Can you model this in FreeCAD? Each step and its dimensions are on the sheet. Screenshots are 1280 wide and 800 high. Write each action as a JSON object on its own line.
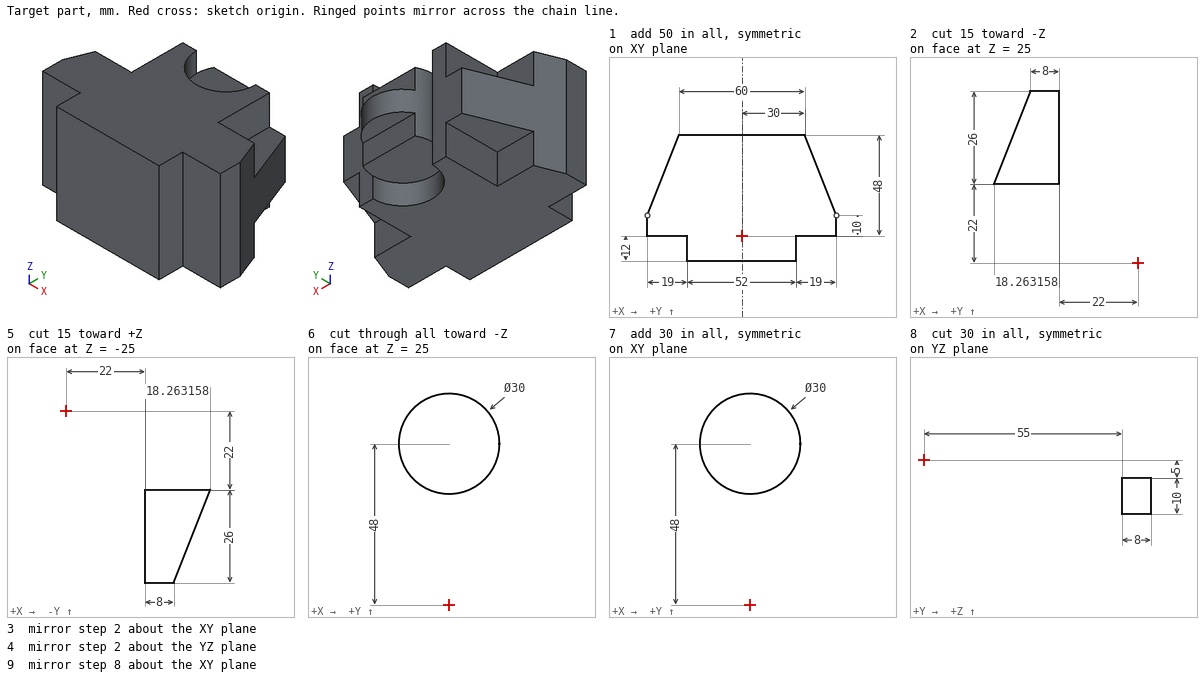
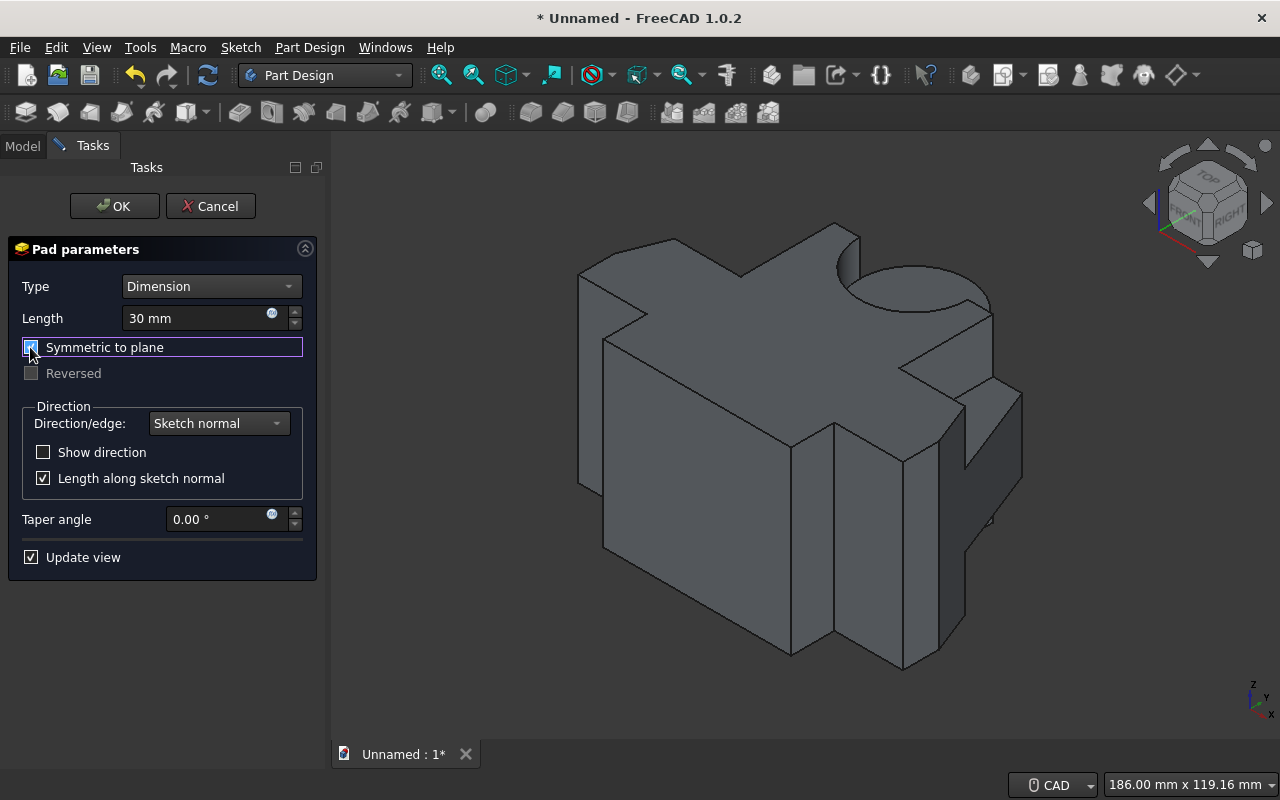
{"action": "left_click", "coordinate": [115, 206]}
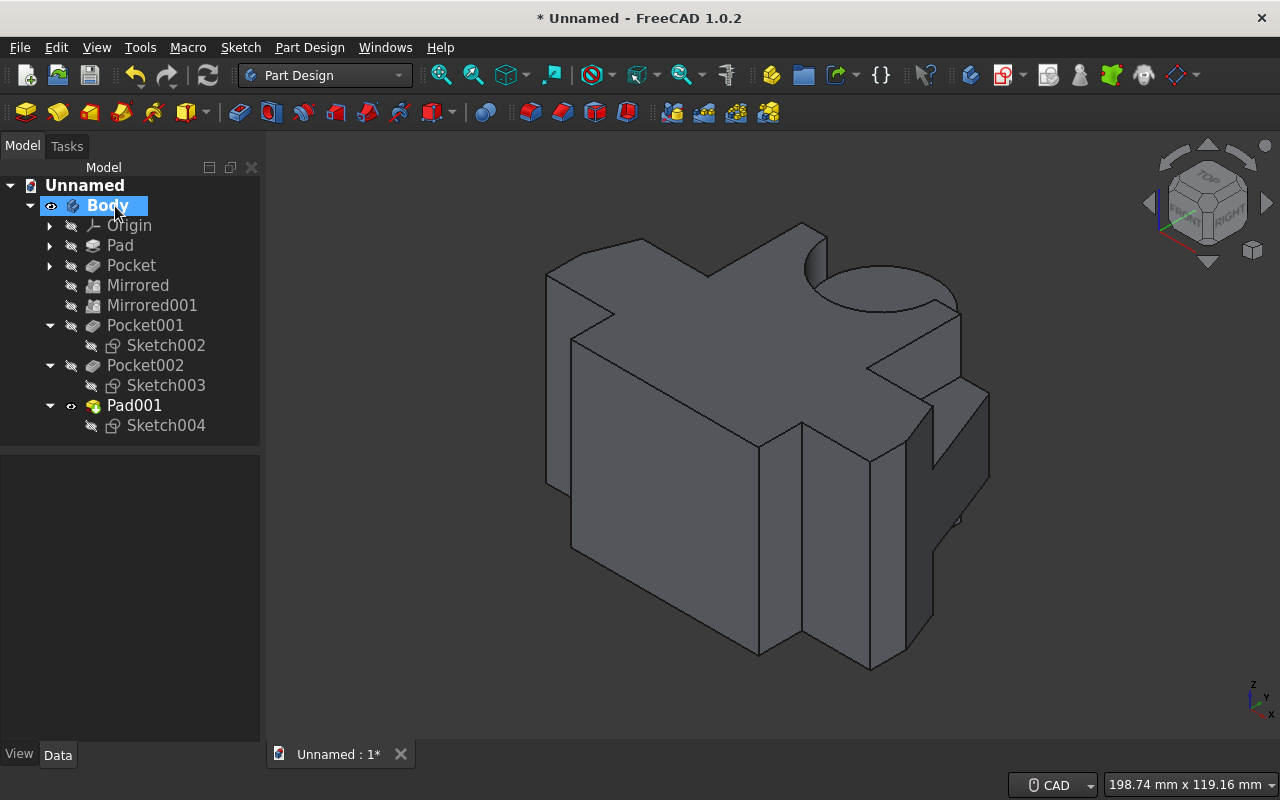
{"action": "left_click", "coordinate": [1004, 76]}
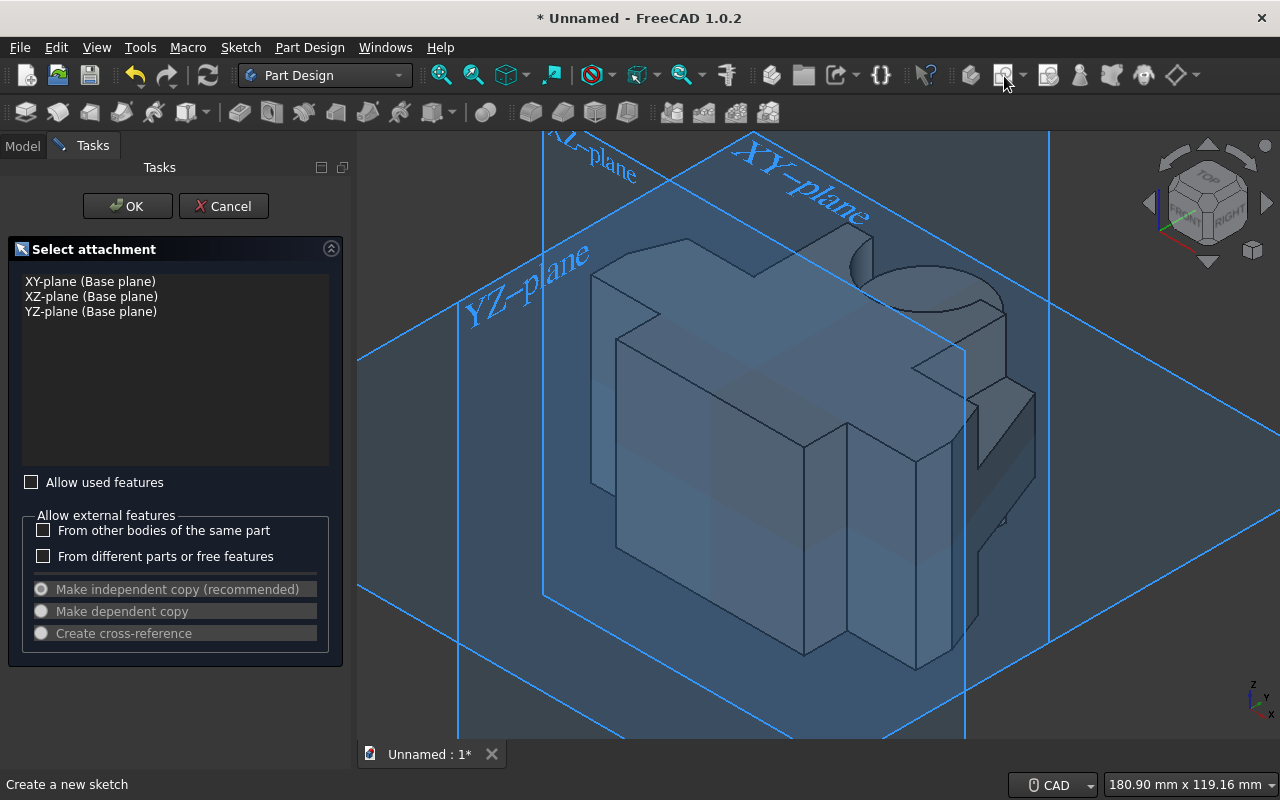
{"action": "left_click", "coordinate": [82, 312]}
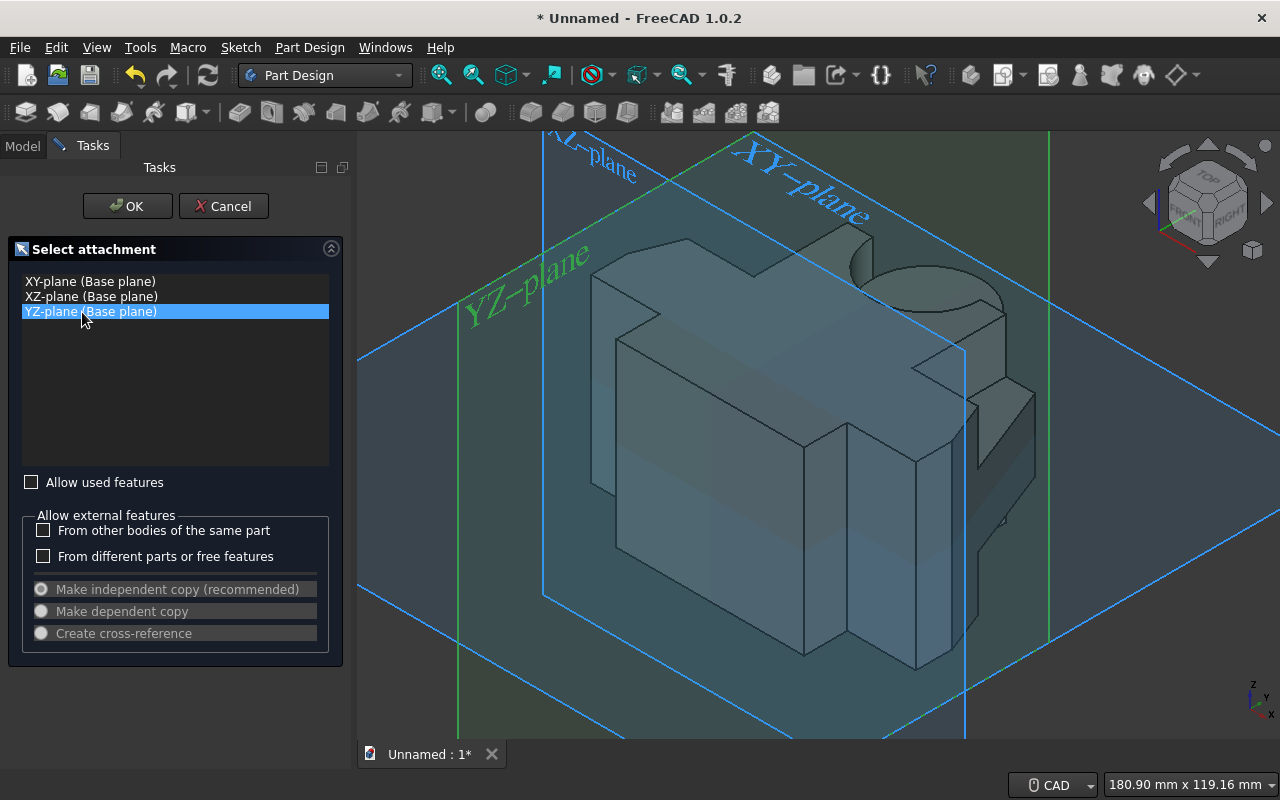
{"action": "left_click", "coordinate": [128, 206]}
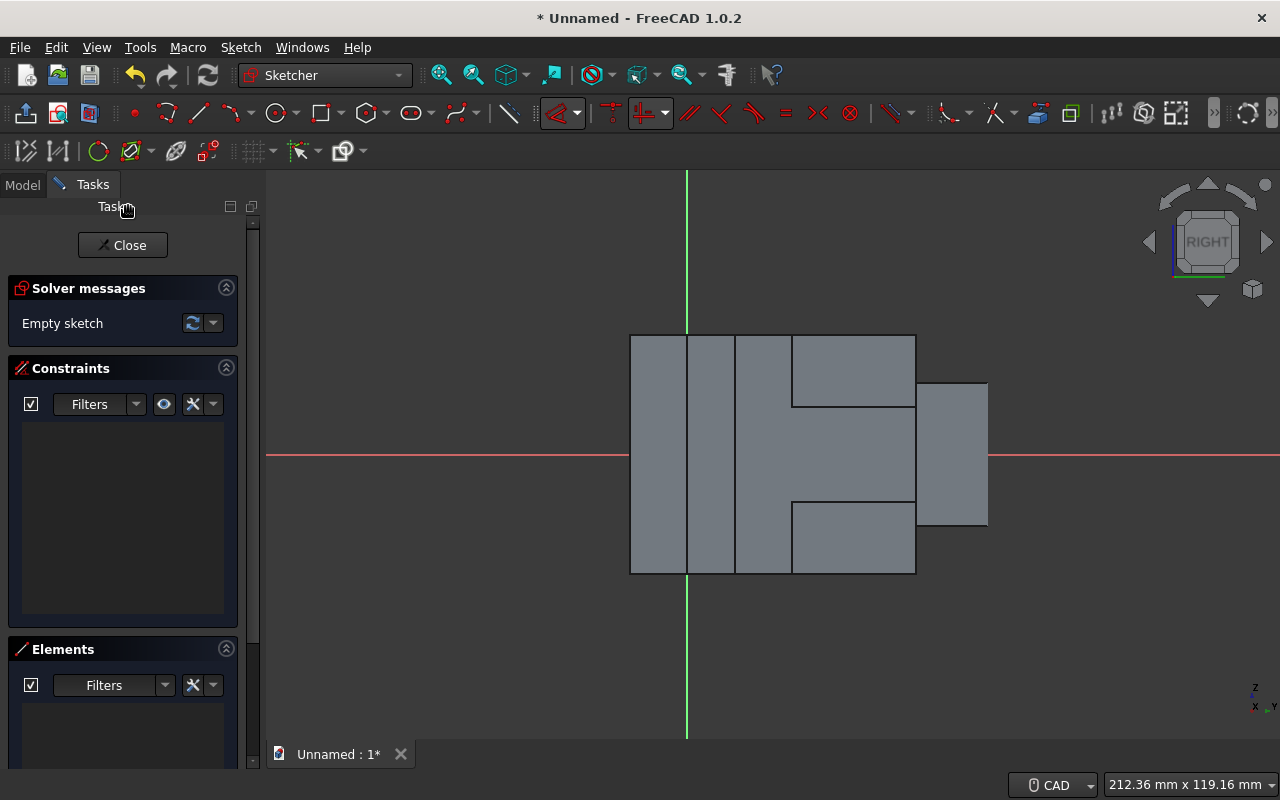
{"action": "left_click", "coordinate": [90, 114]}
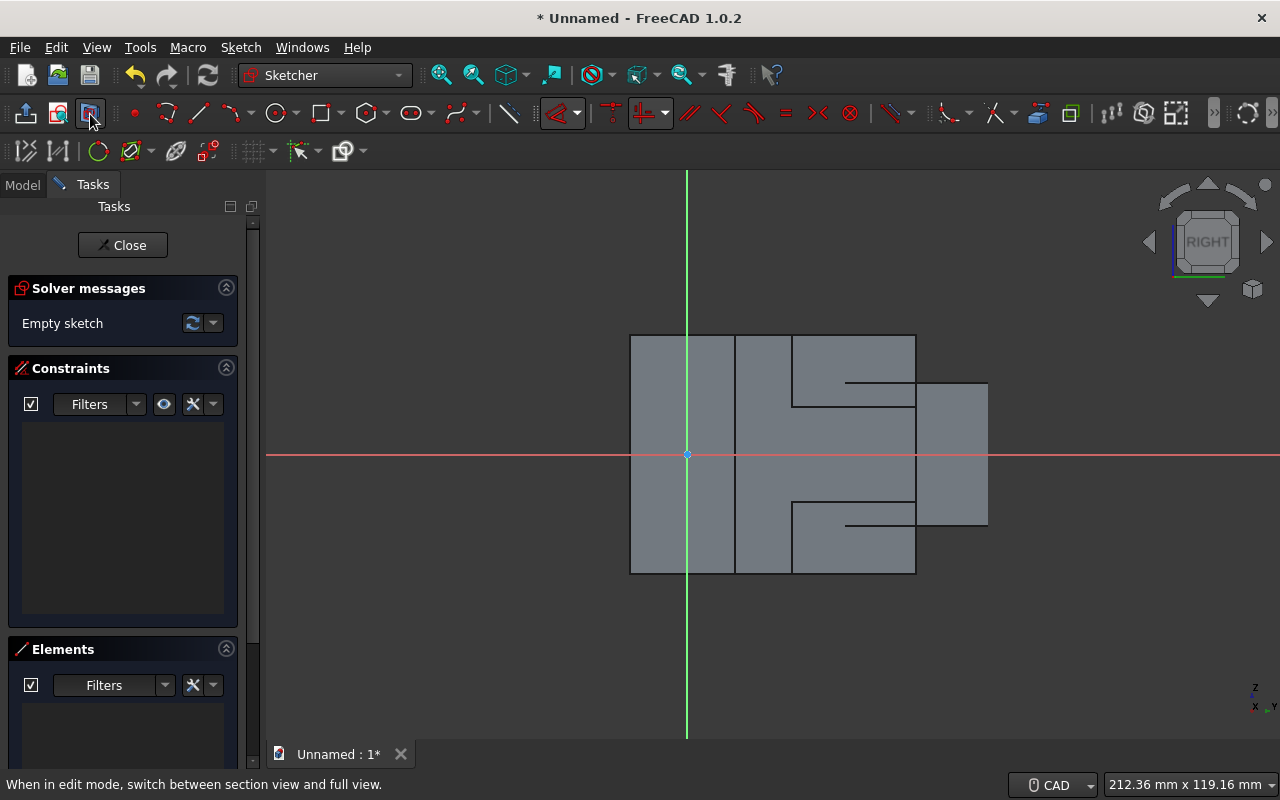
{"action": "scroll", "coordinate": [1010, 510], "scroll_direction": "up", "scroll_amount": 10}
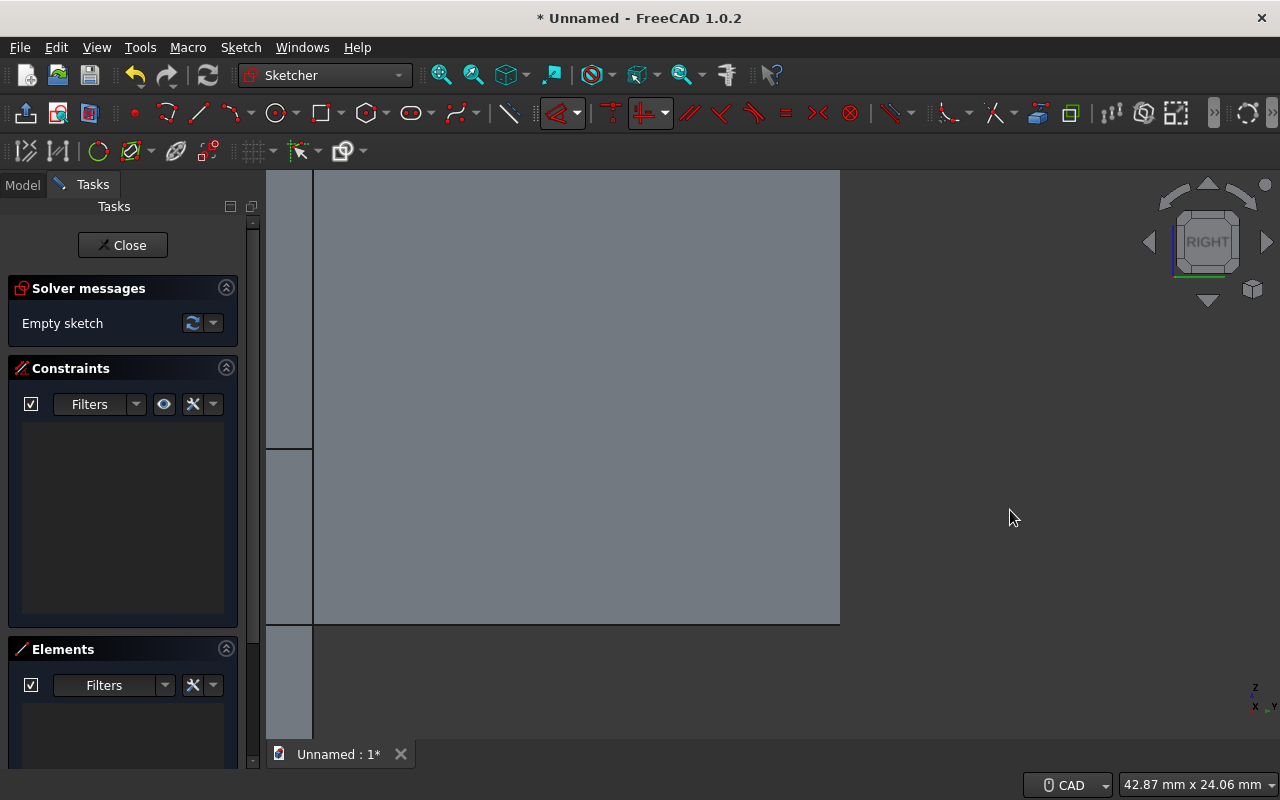
{"action": "left_click", "coordinate": [322, 114]}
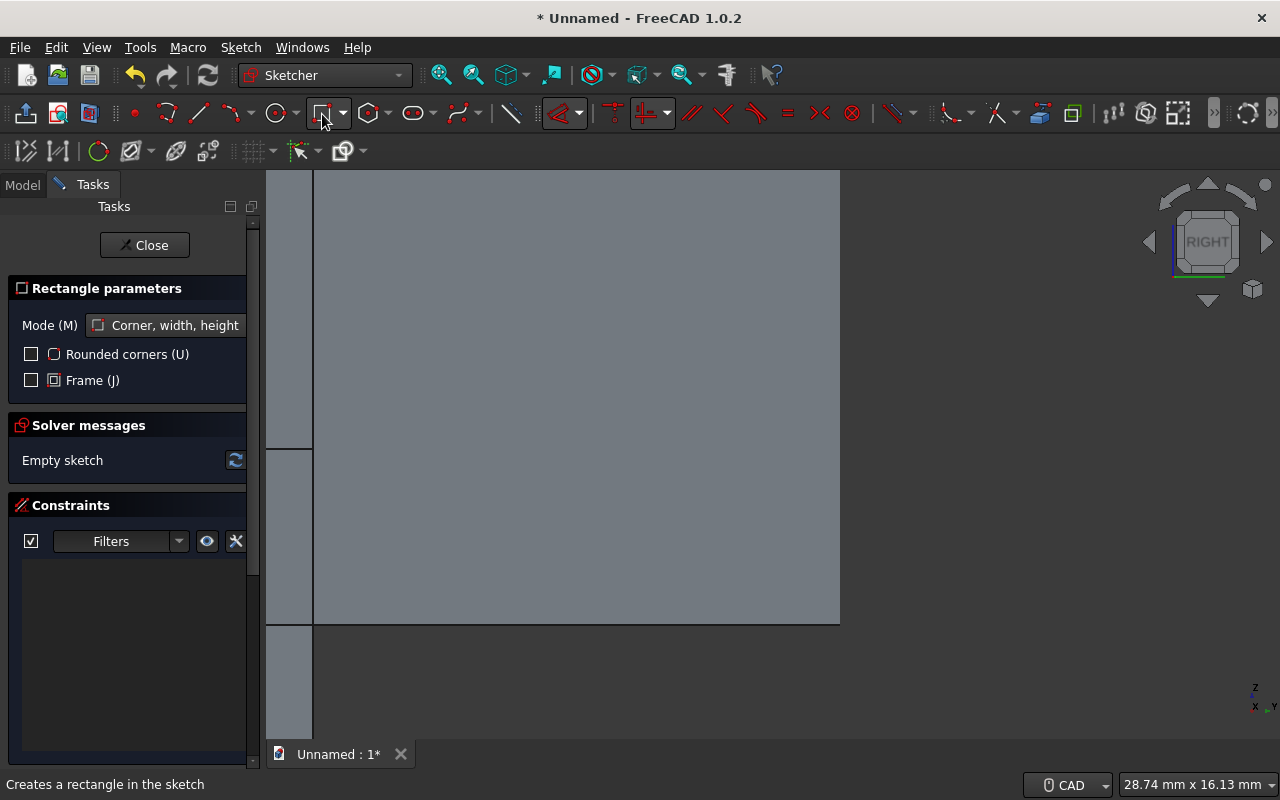
{"action": "left_click", "coordinate": [560, 272]}
{"action": "left_click", "coordinate": [842, 625]}
{"action": "key", "text": "Escape"}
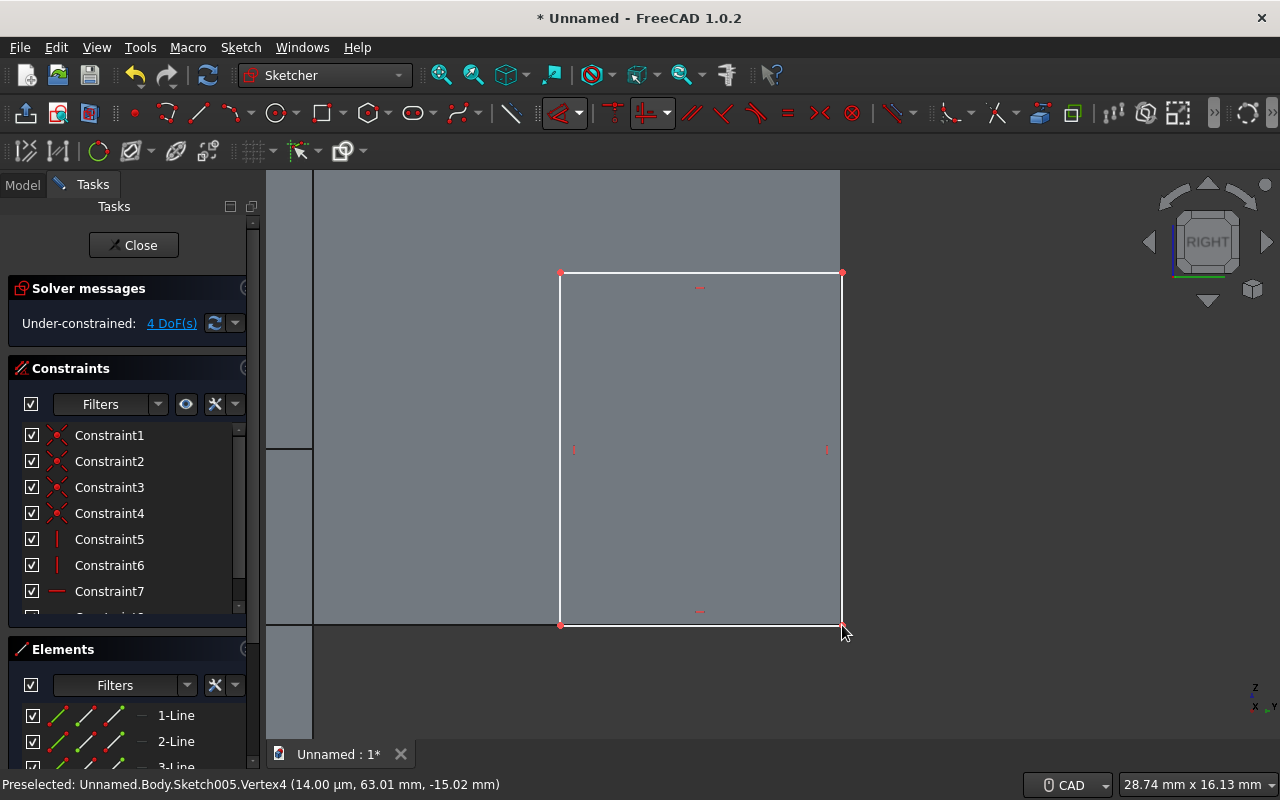
{"action": "left_click", "coordinate": [645, 626]}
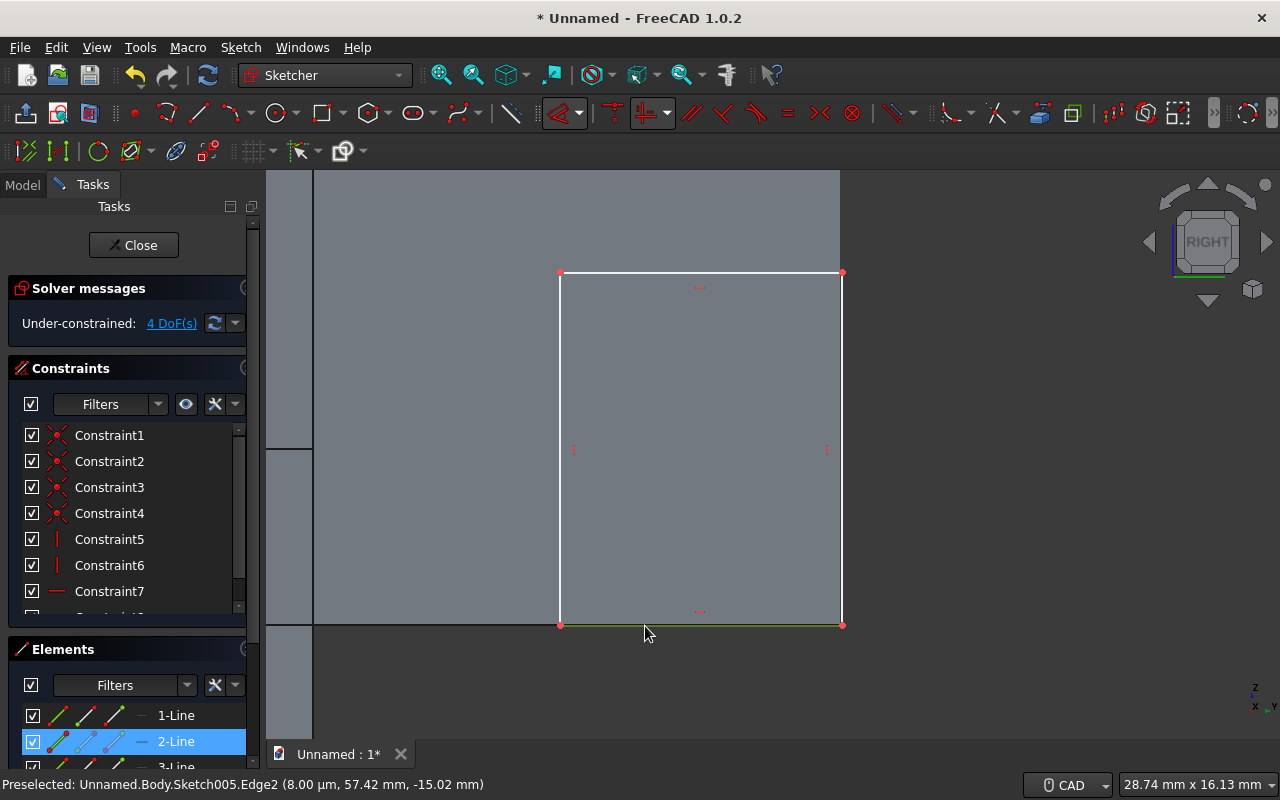
{"action": "left_click", "coordinate": [582, 114]}